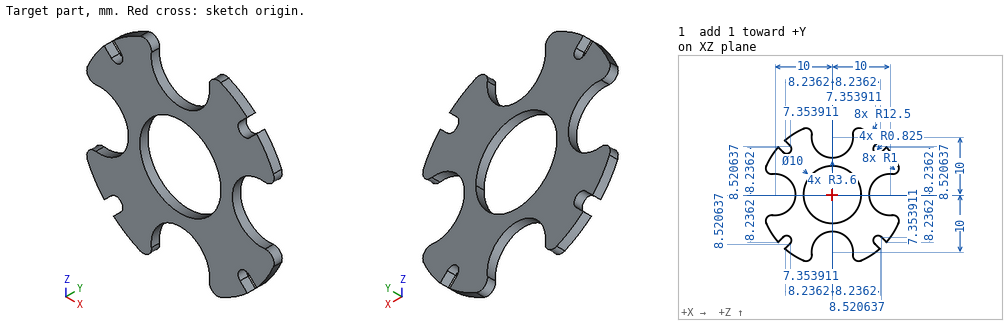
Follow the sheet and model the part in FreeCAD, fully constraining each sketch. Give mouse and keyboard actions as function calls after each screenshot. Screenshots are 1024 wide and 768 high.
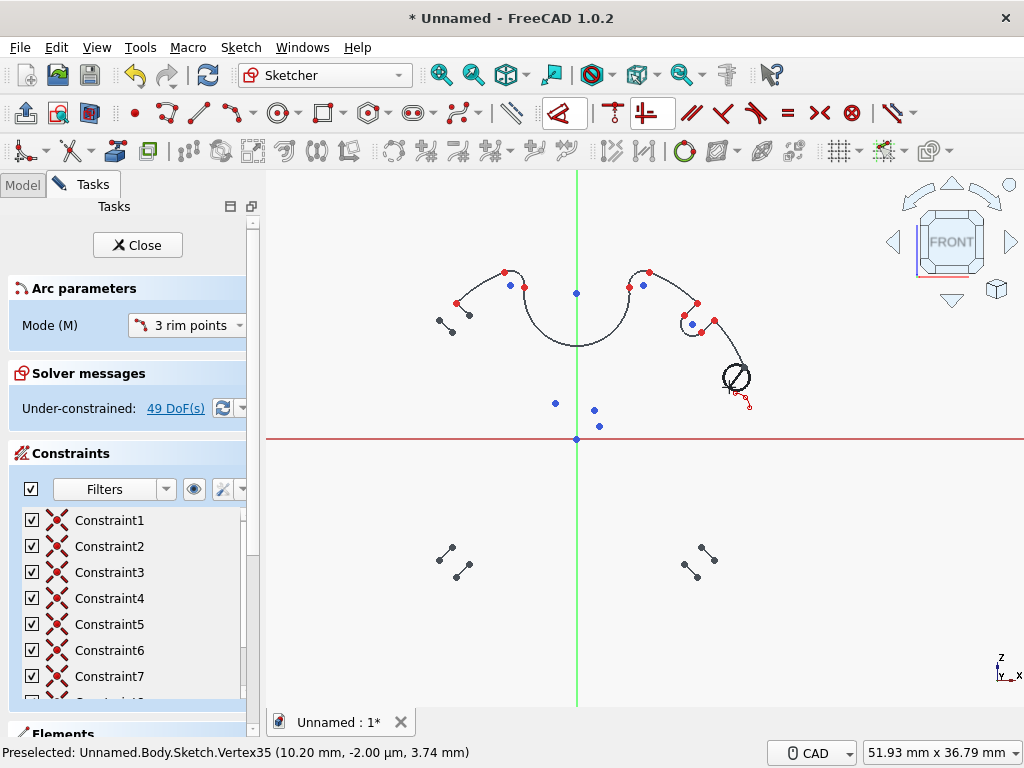
scroll(743, 381, up, 4)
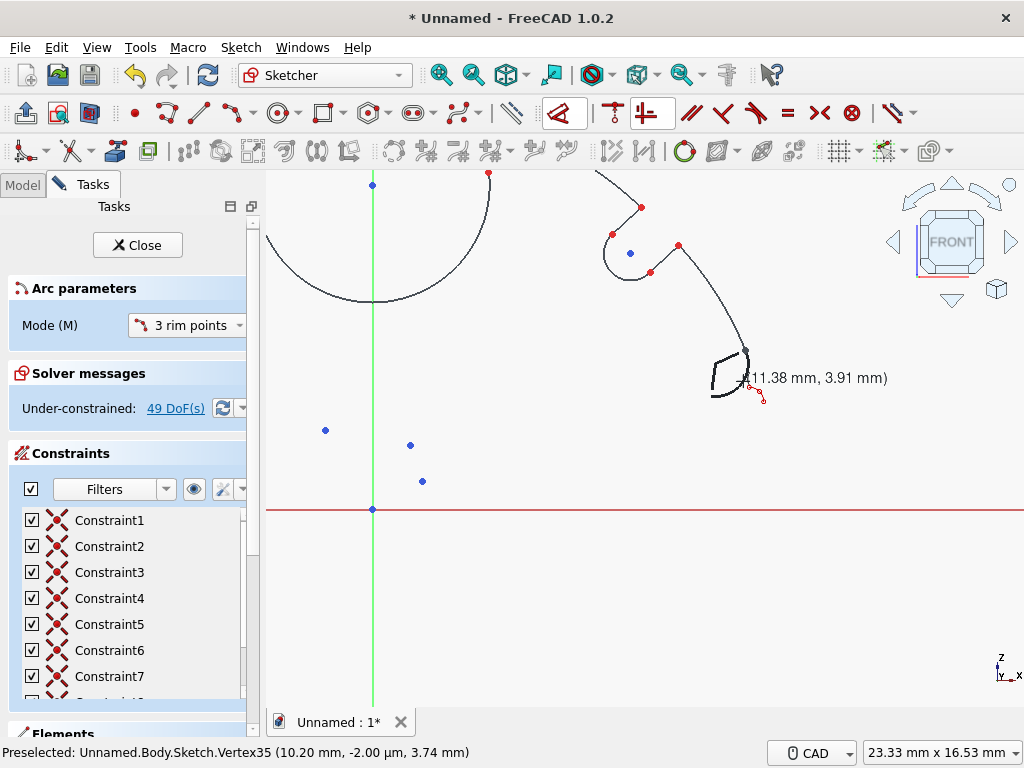
click(741, 381)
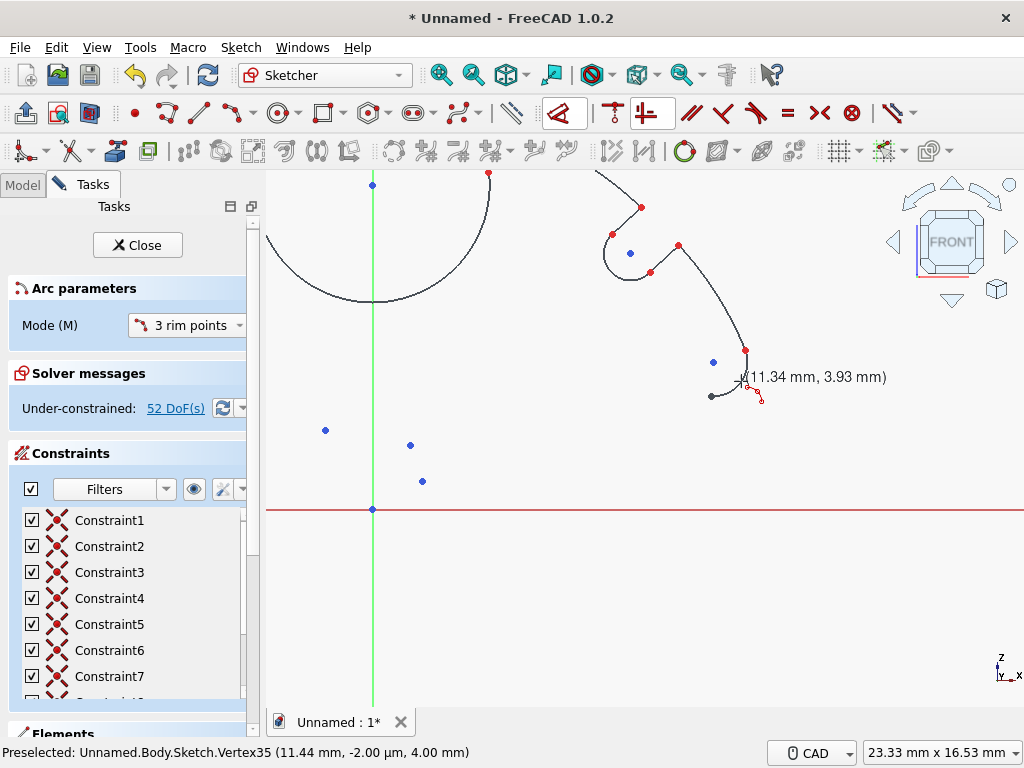
click(711, 396)
click(712, 626)
click(587, 471)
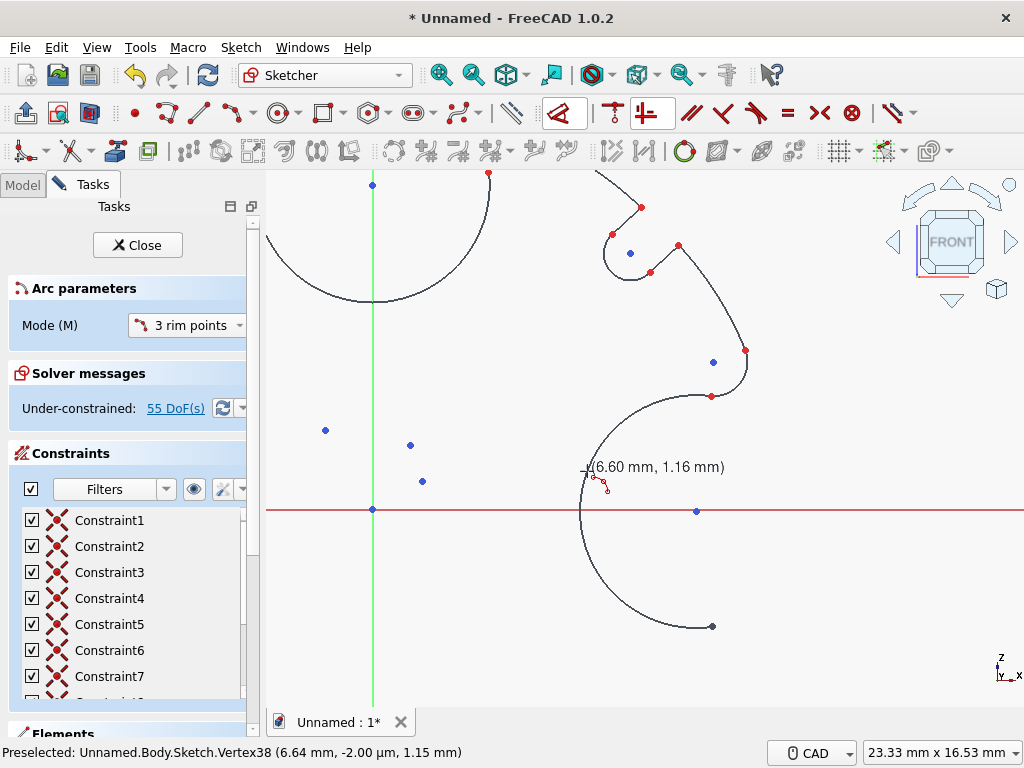
click(712, 627)
click(745, 671)
click(741, 639)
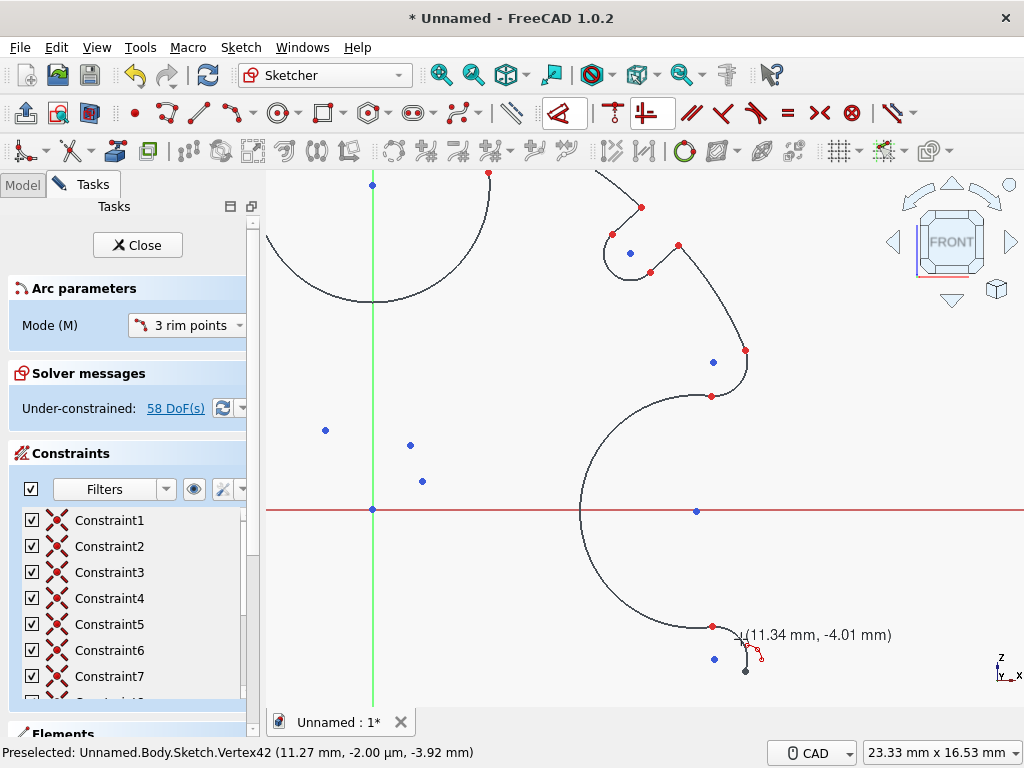
click(745, 672)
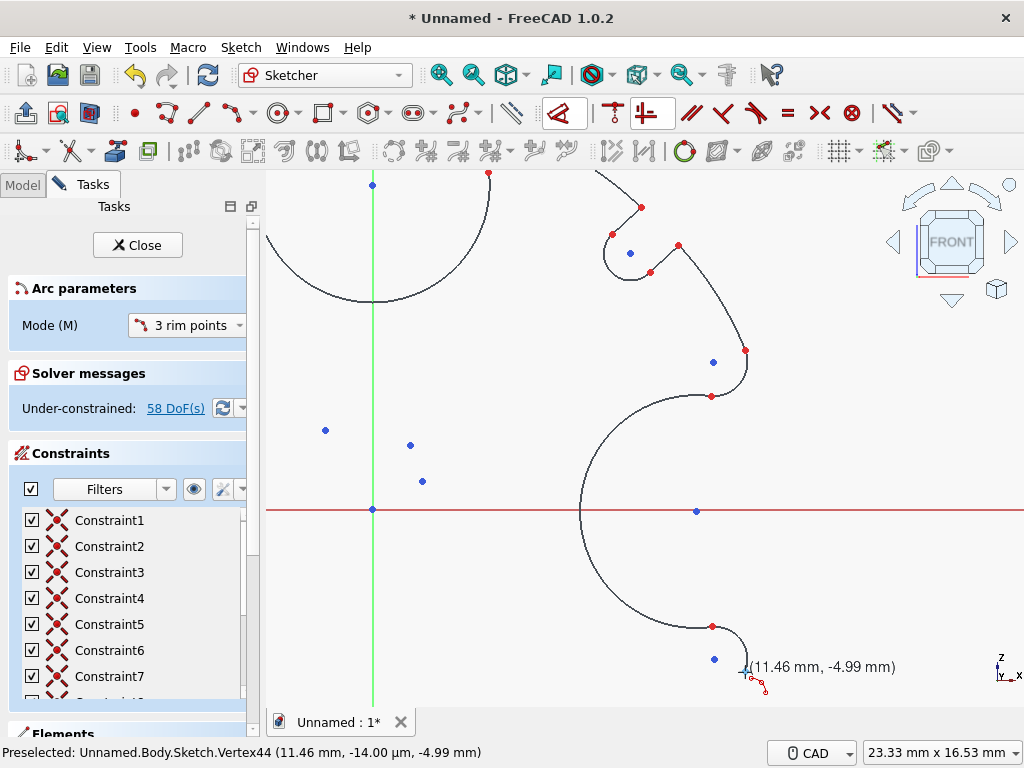
scroll(743, 380, down, 4)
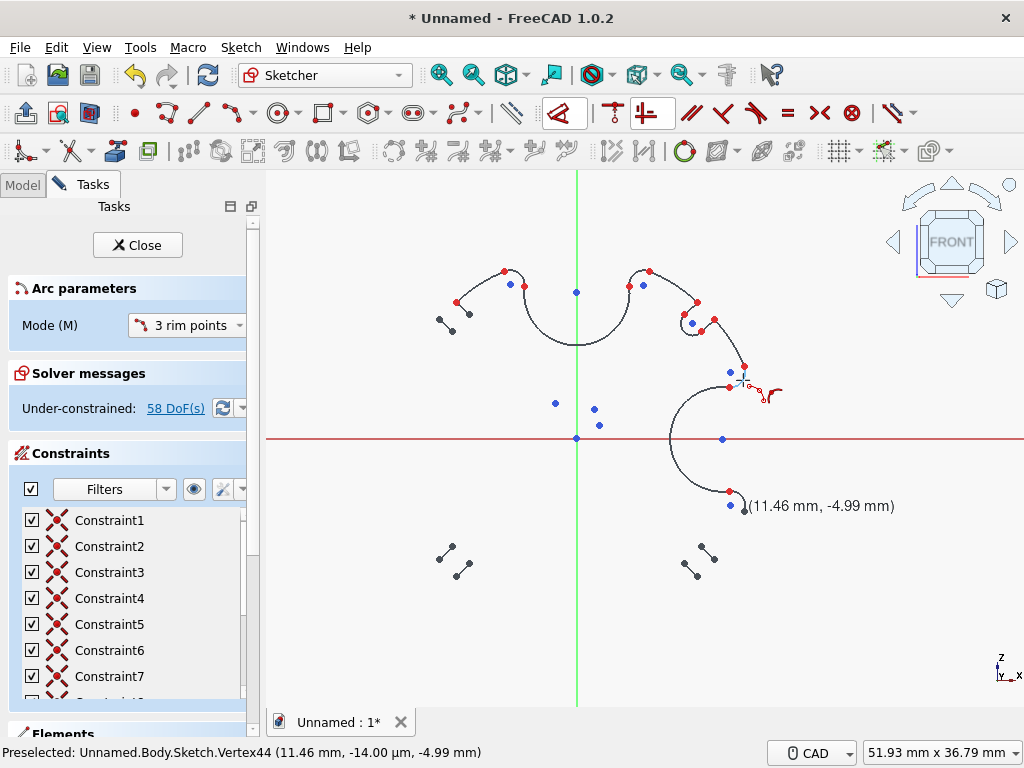
scroll(714, 559, up, 3)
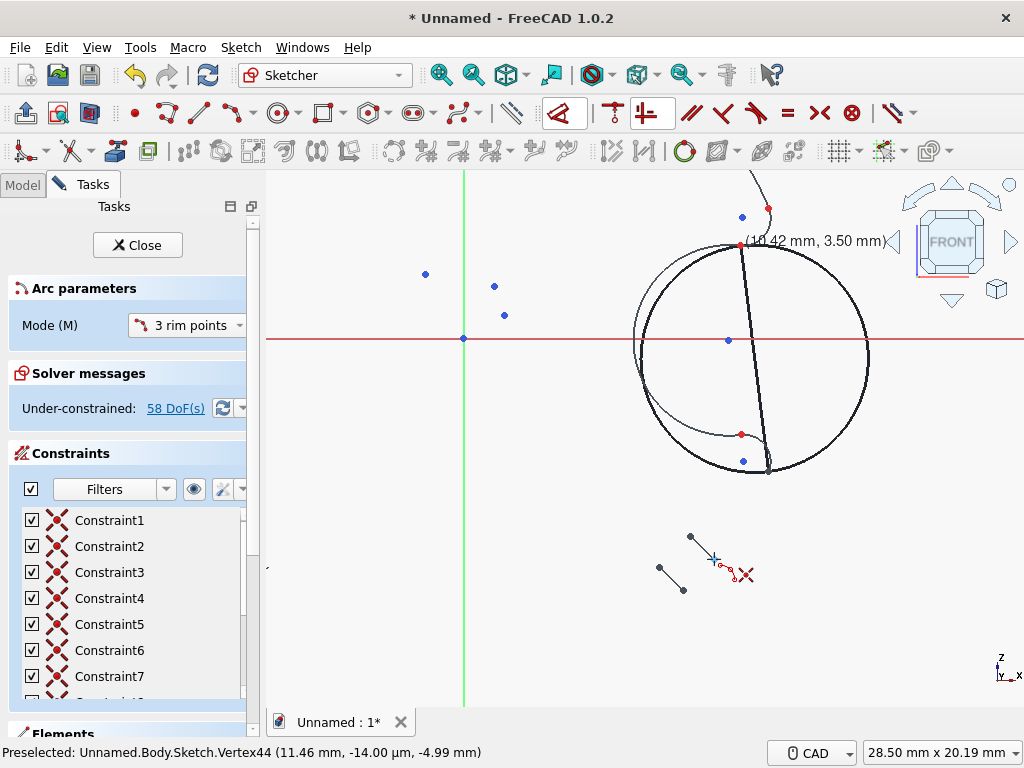
click(715, 560)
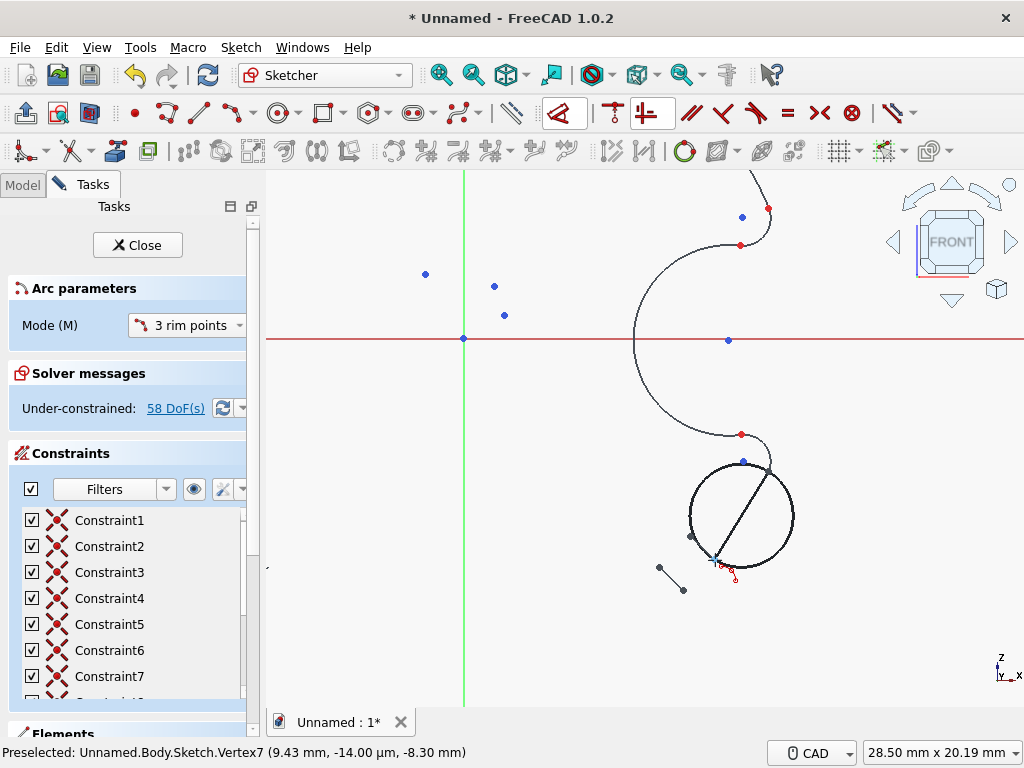
scroll(745, 517, up, 7)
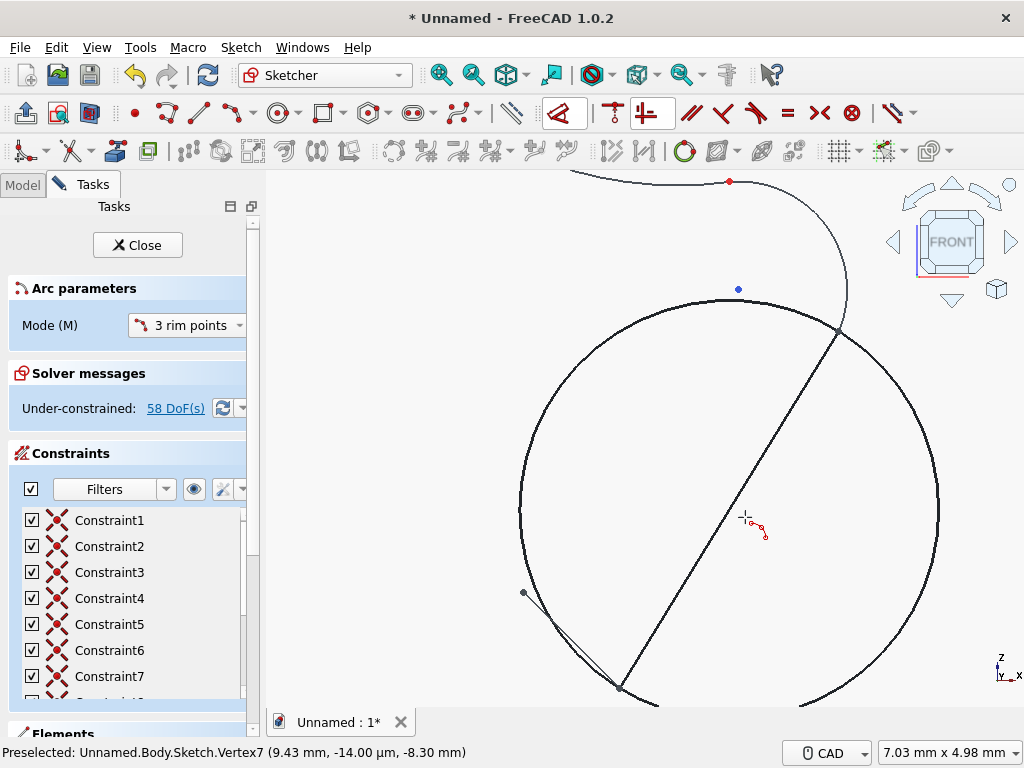
click(742, 513)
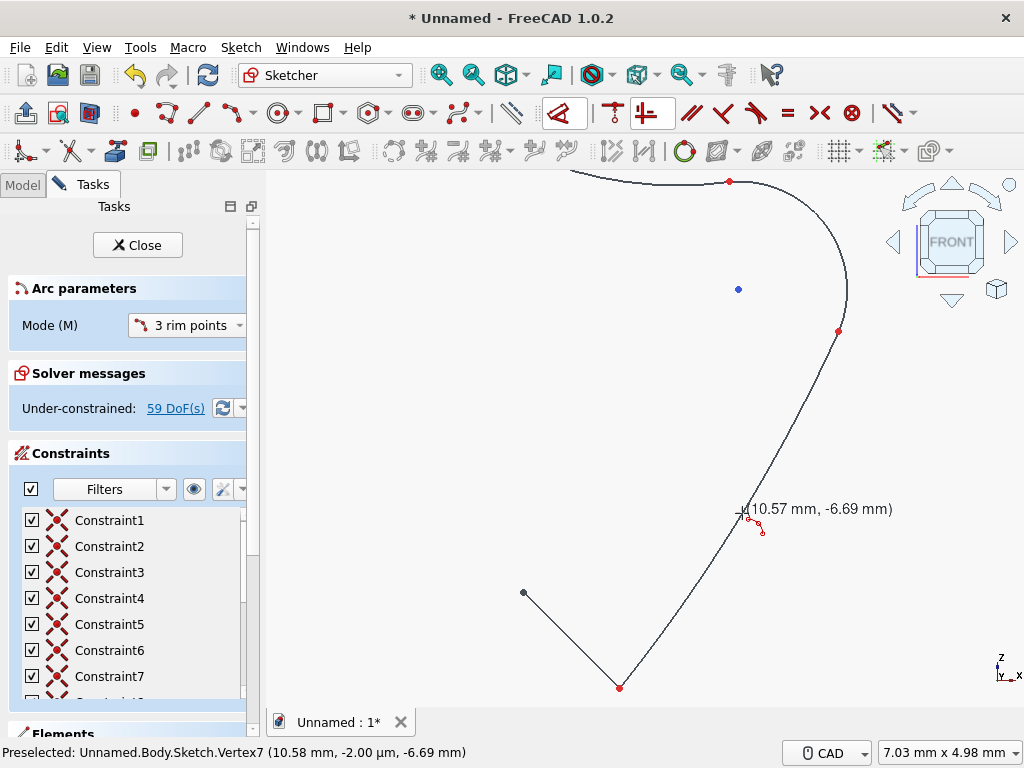
scroll(729, 540, down, 10)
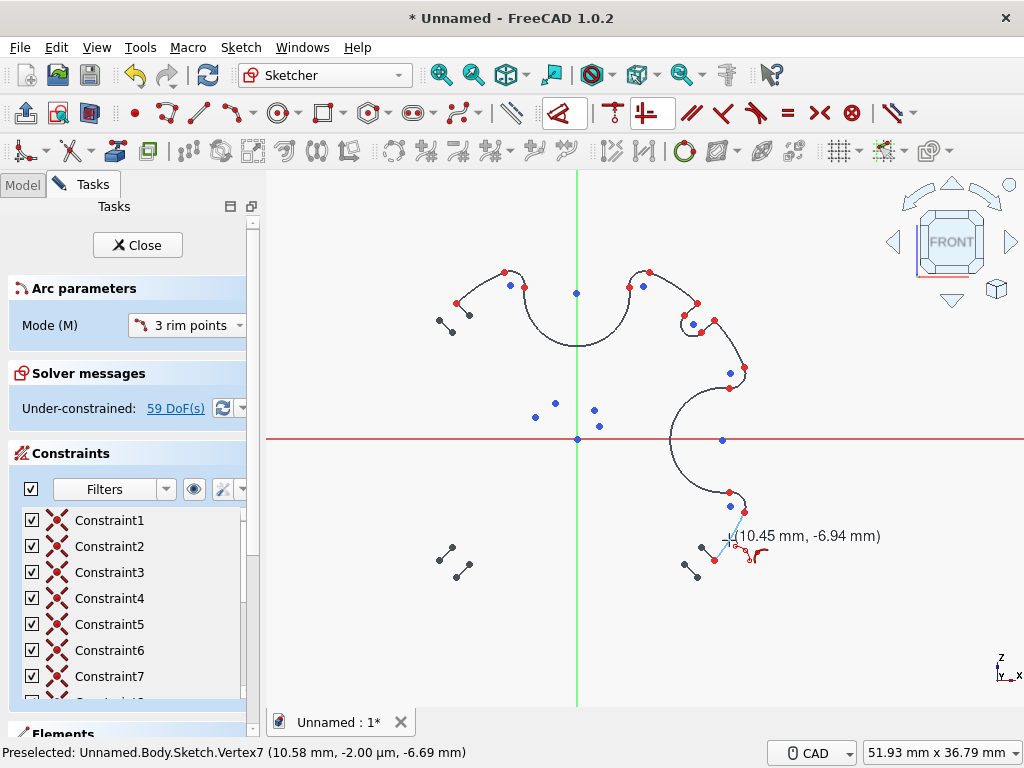
scroll(701, 547, up, 3)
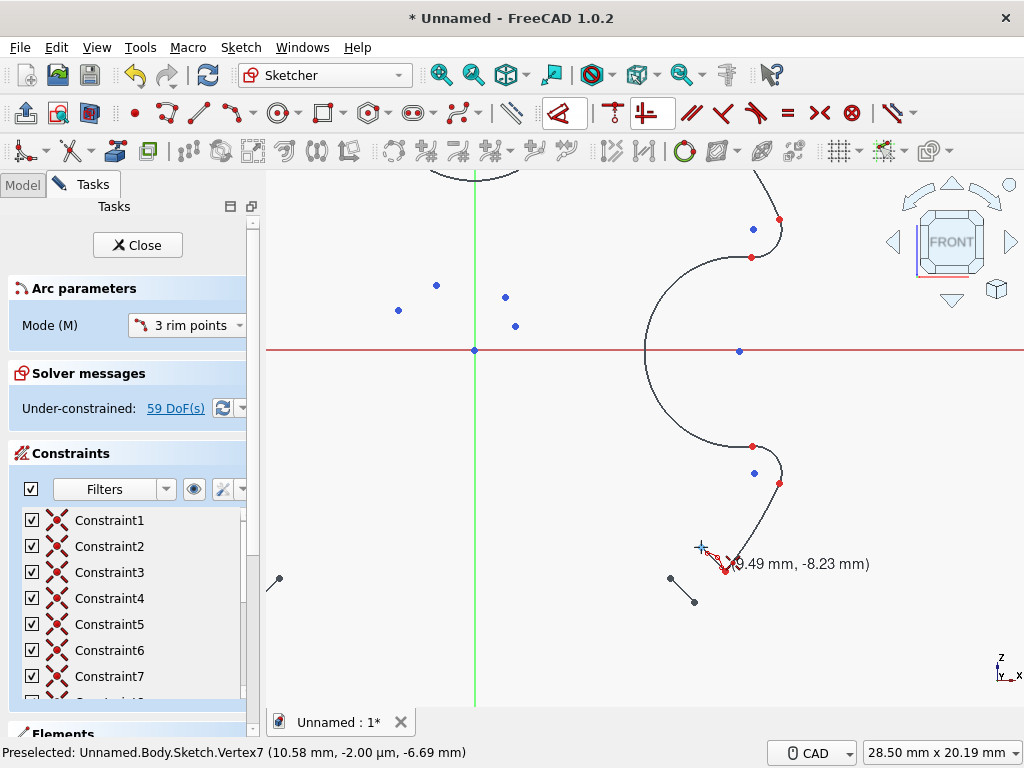
click(702, 548)
click(671, 579)
click(670, 546)